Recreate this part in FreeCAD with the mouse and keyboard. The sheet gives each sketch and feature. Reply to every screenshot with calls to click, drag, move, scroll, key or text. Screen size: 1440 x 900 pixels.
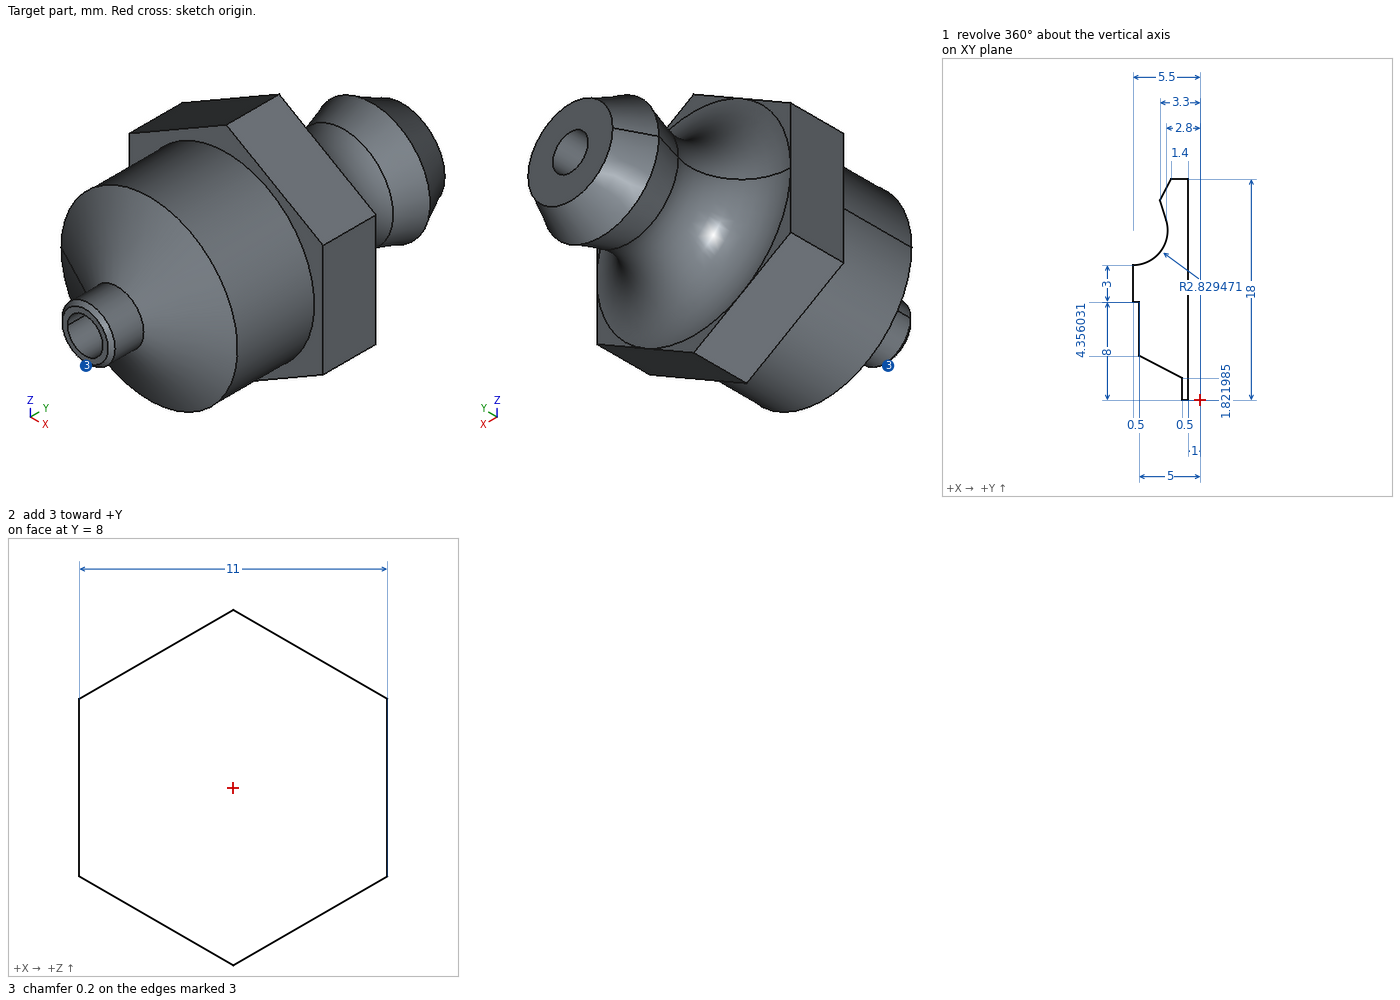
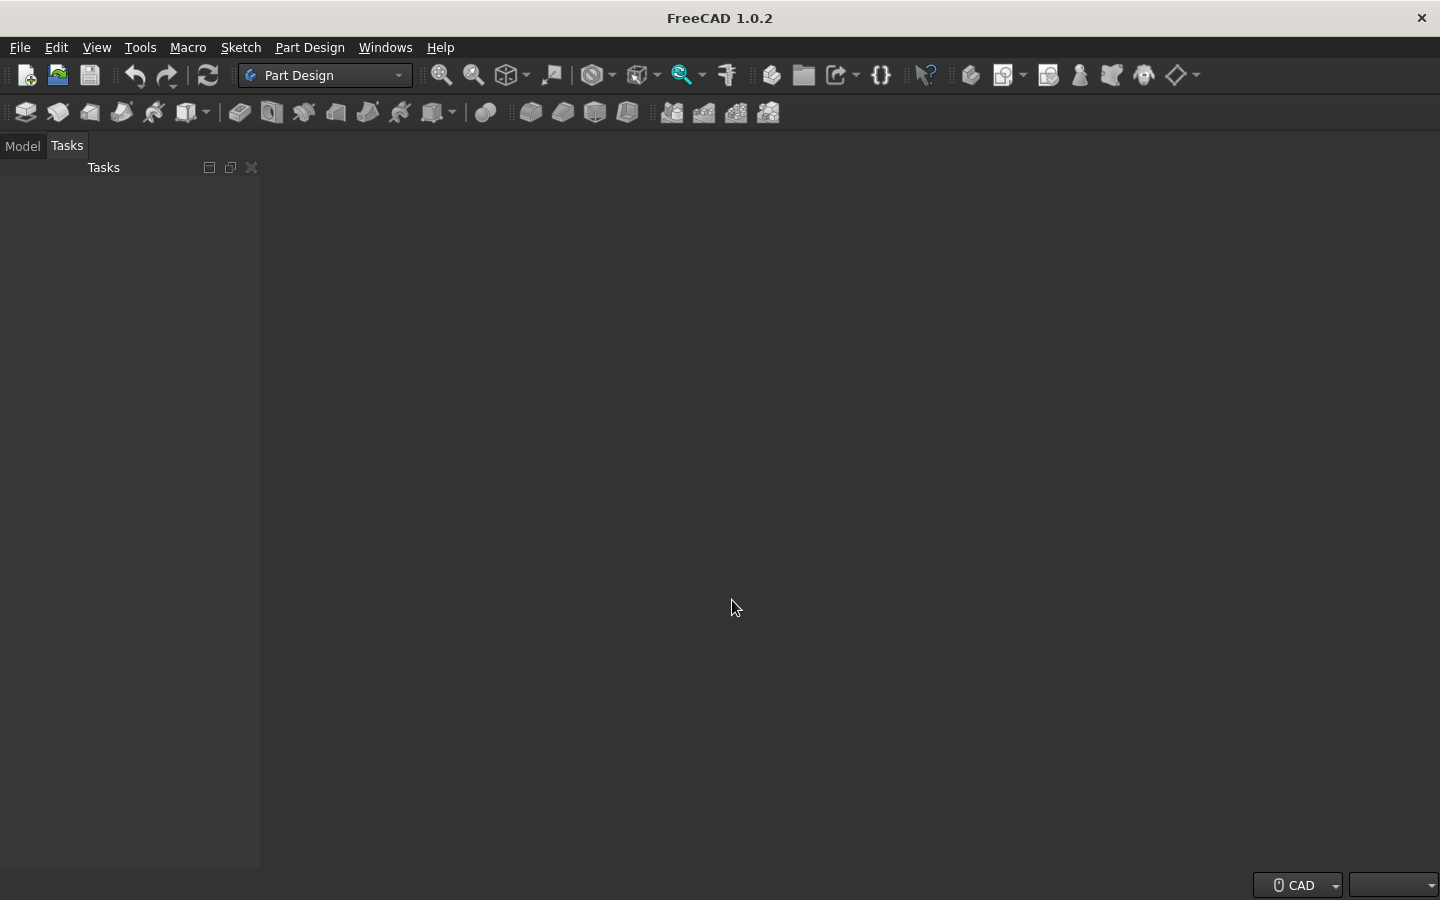
click(26, 76)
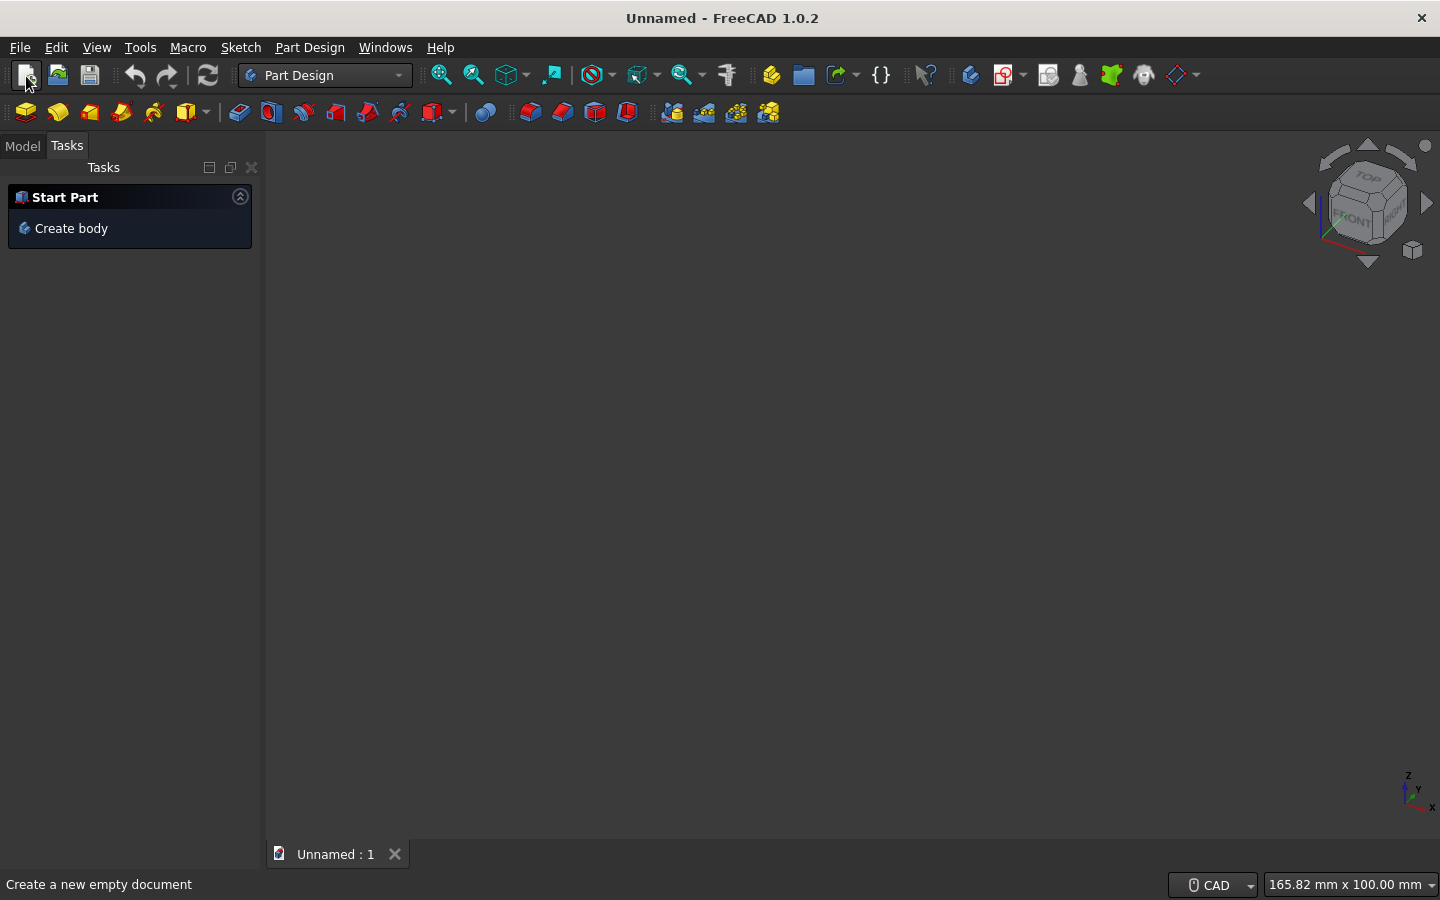
click(1004, 76)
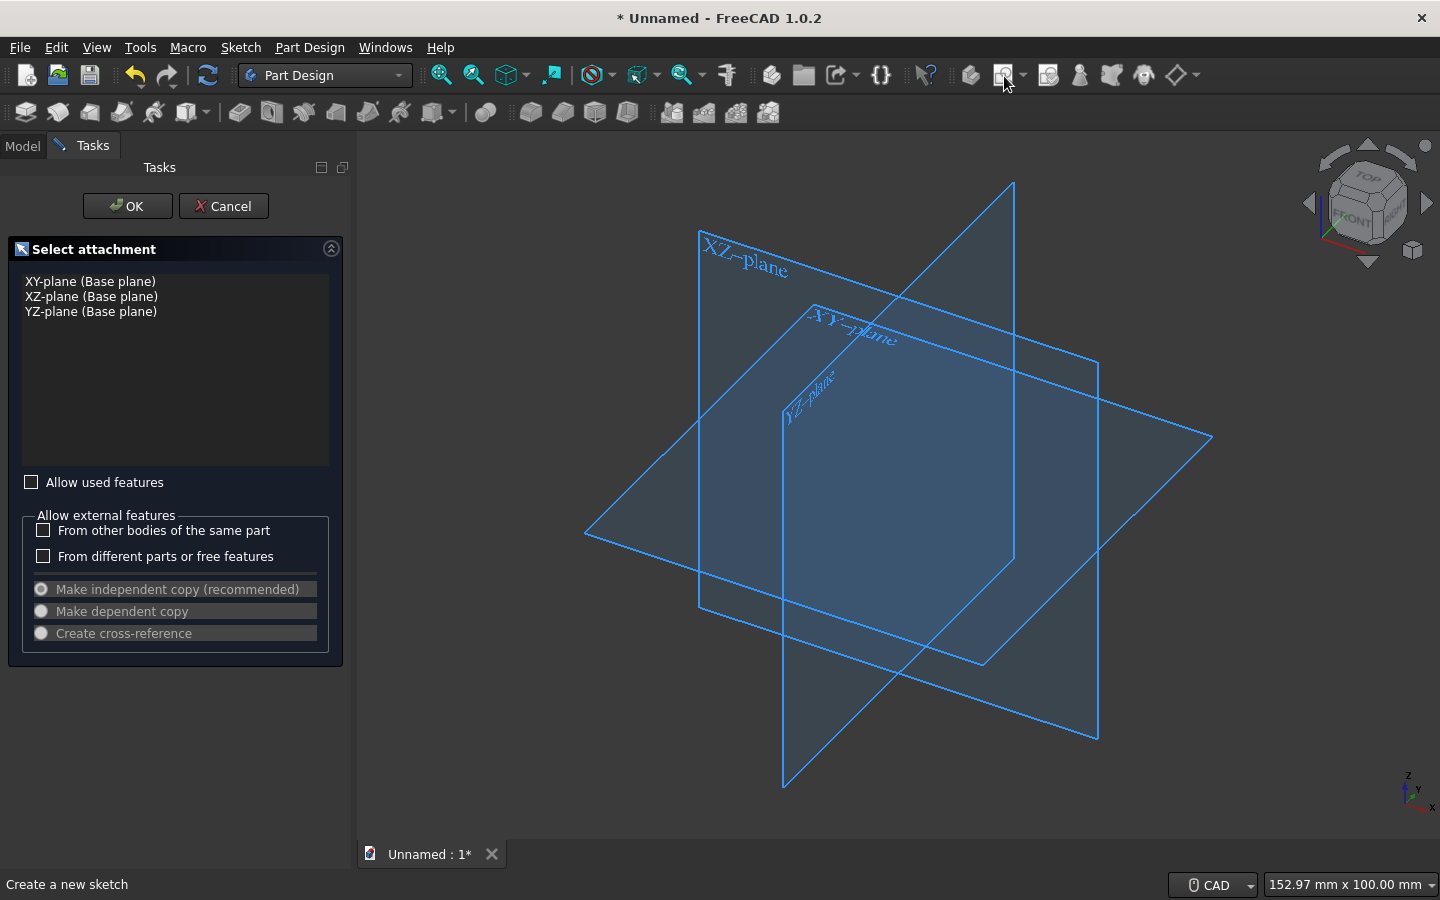
click(82, 282)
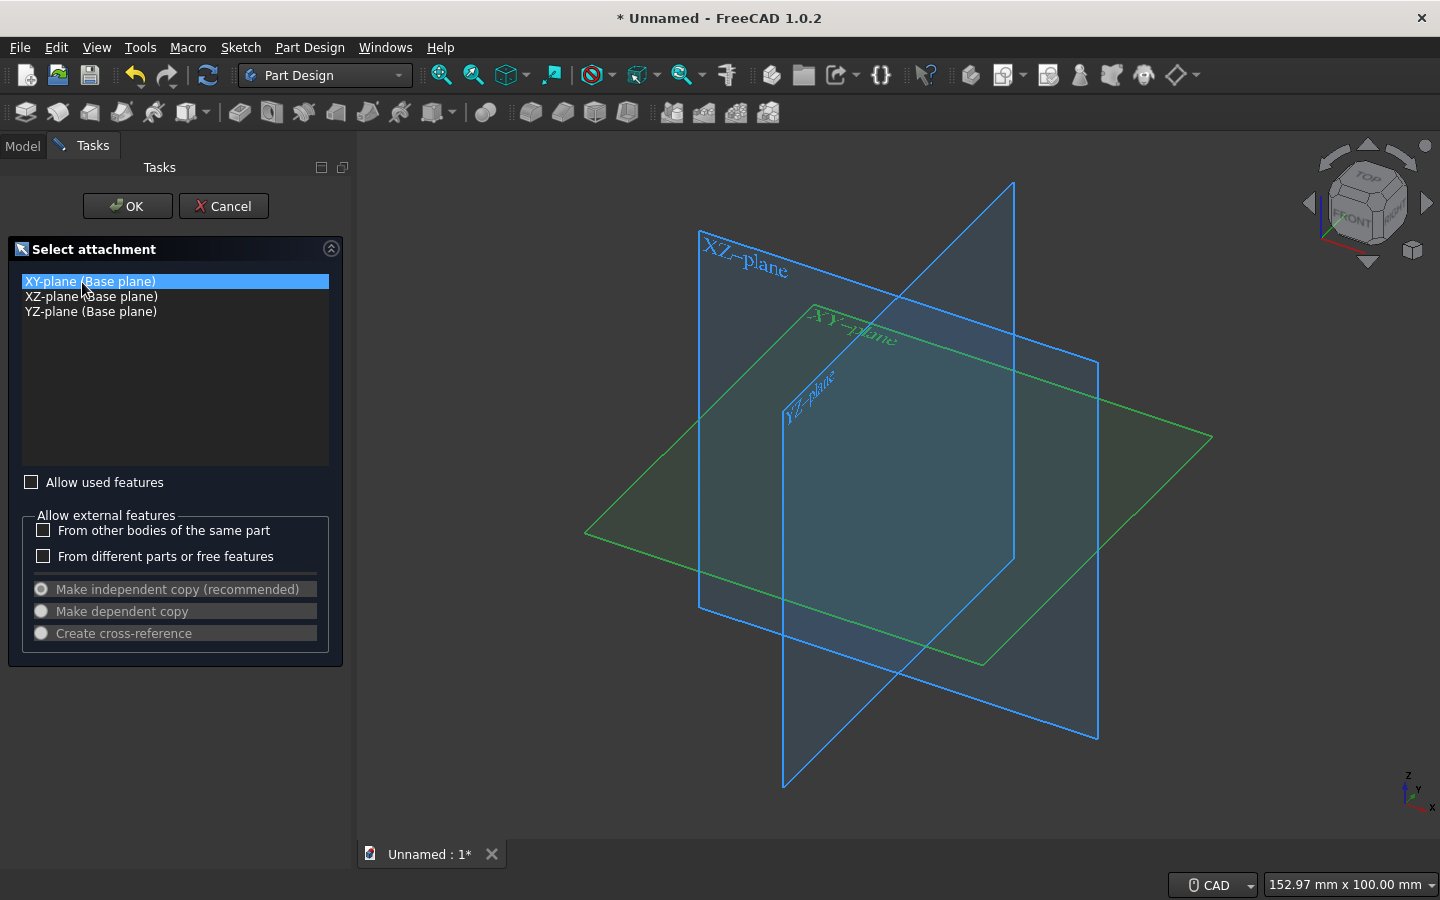
click(128, 206)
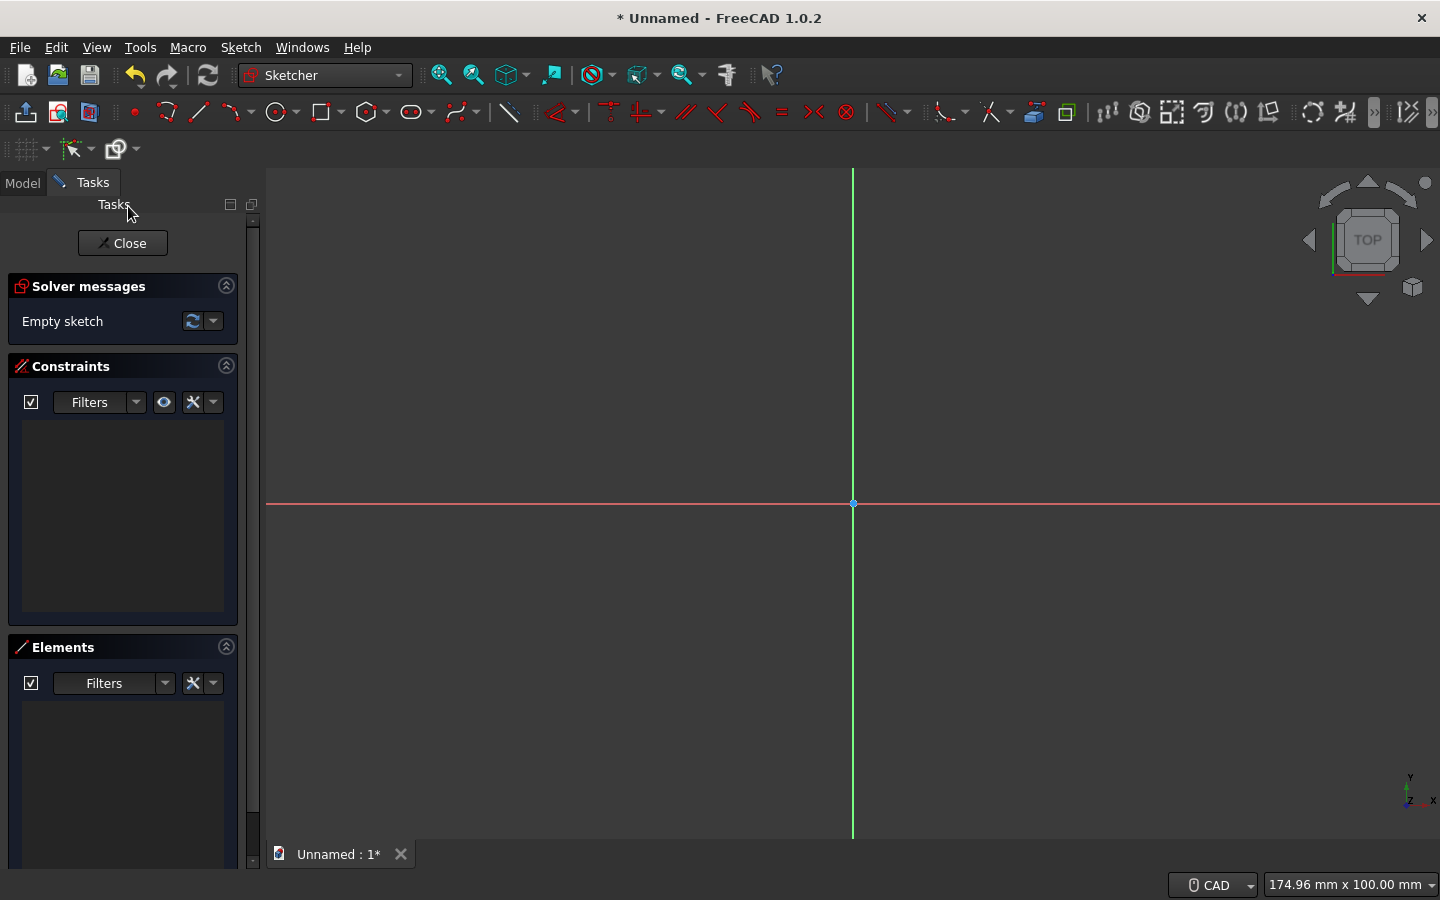
scroll(856, 417, up, 6)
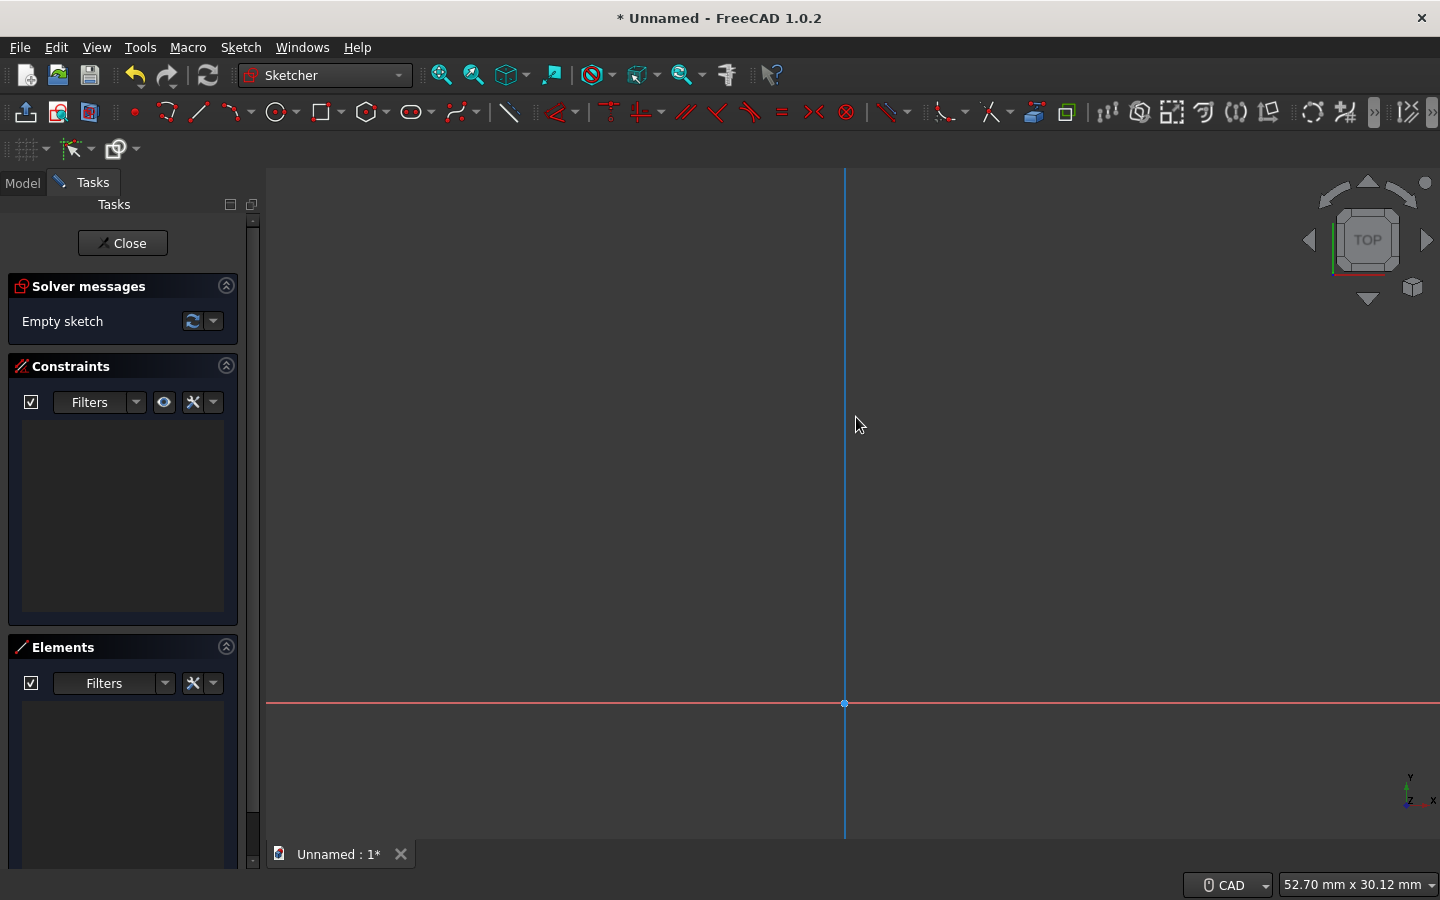
click(168, 112)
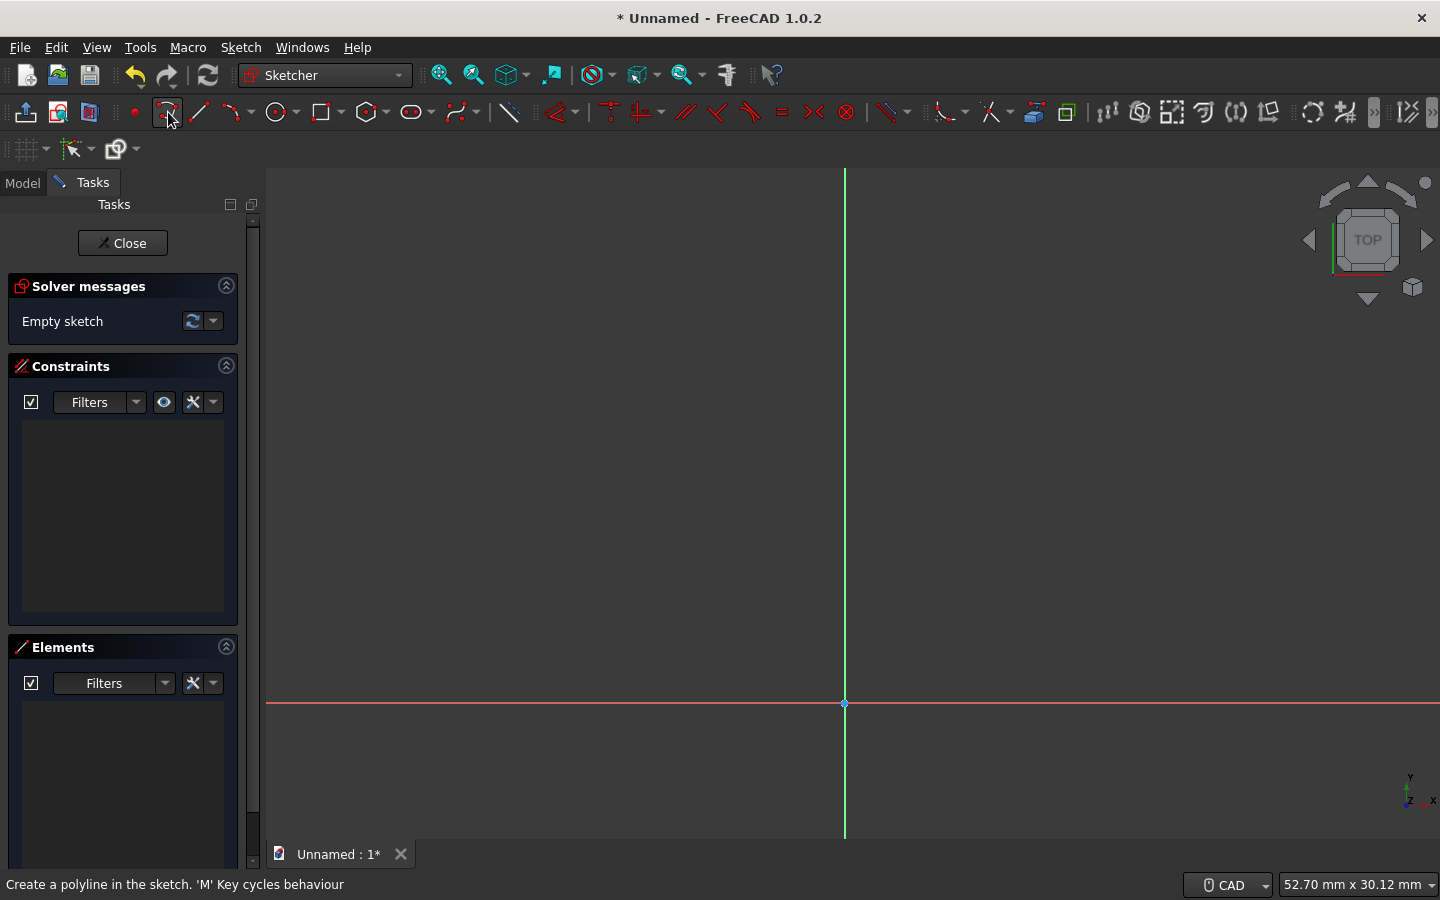
click(722, 458)
click(722, 525)